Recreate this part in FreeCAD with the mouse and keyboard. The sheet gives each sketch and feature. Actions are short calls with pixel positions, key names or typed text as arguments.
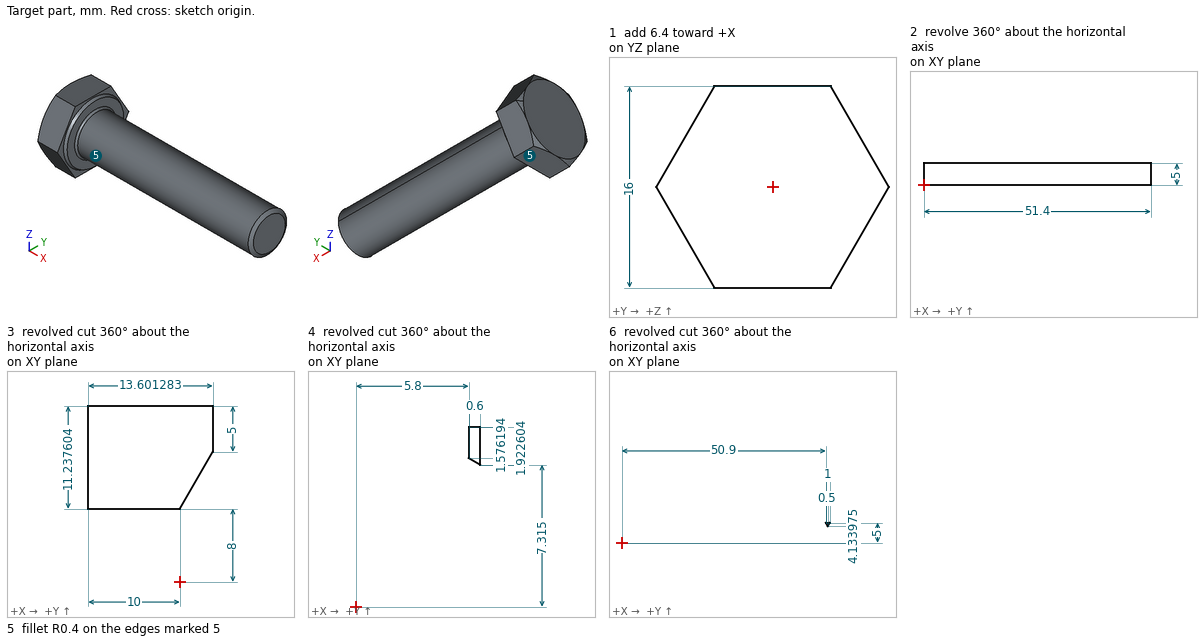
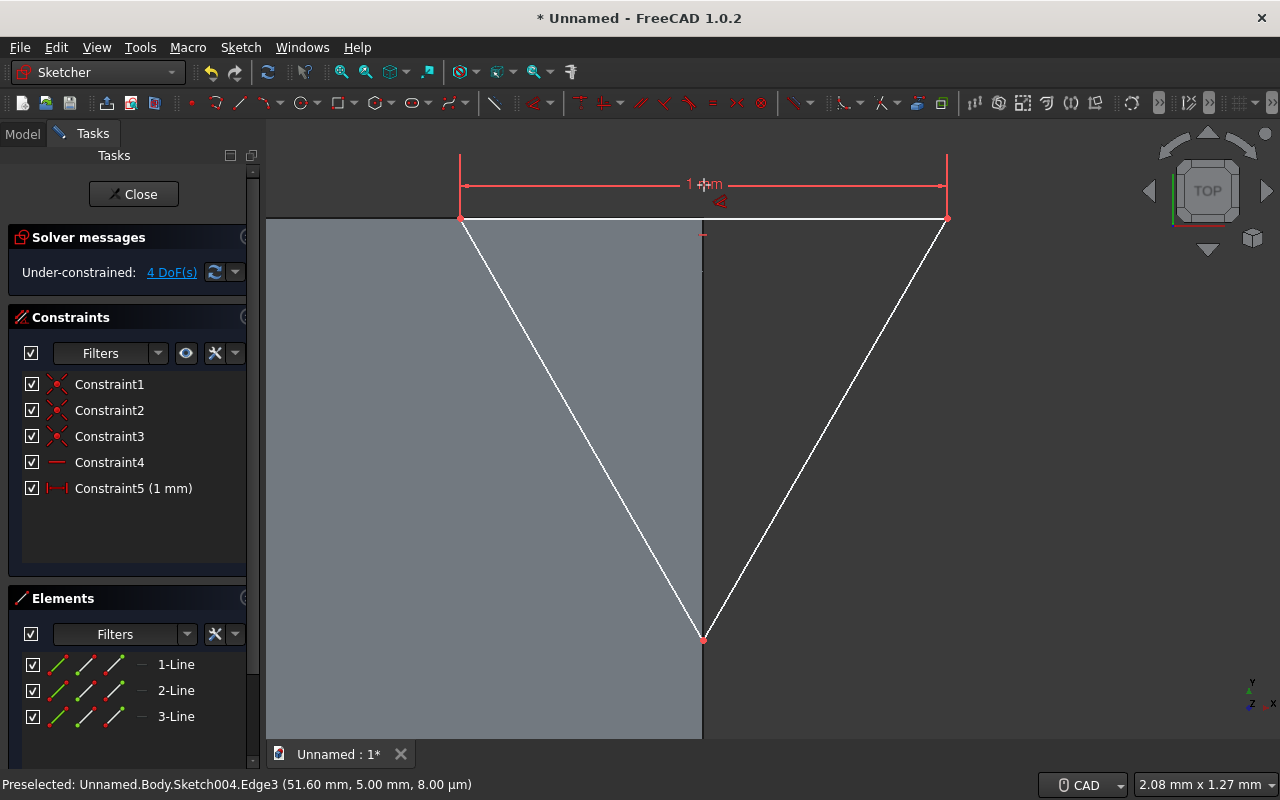
click(460, 219)
click(494, 465)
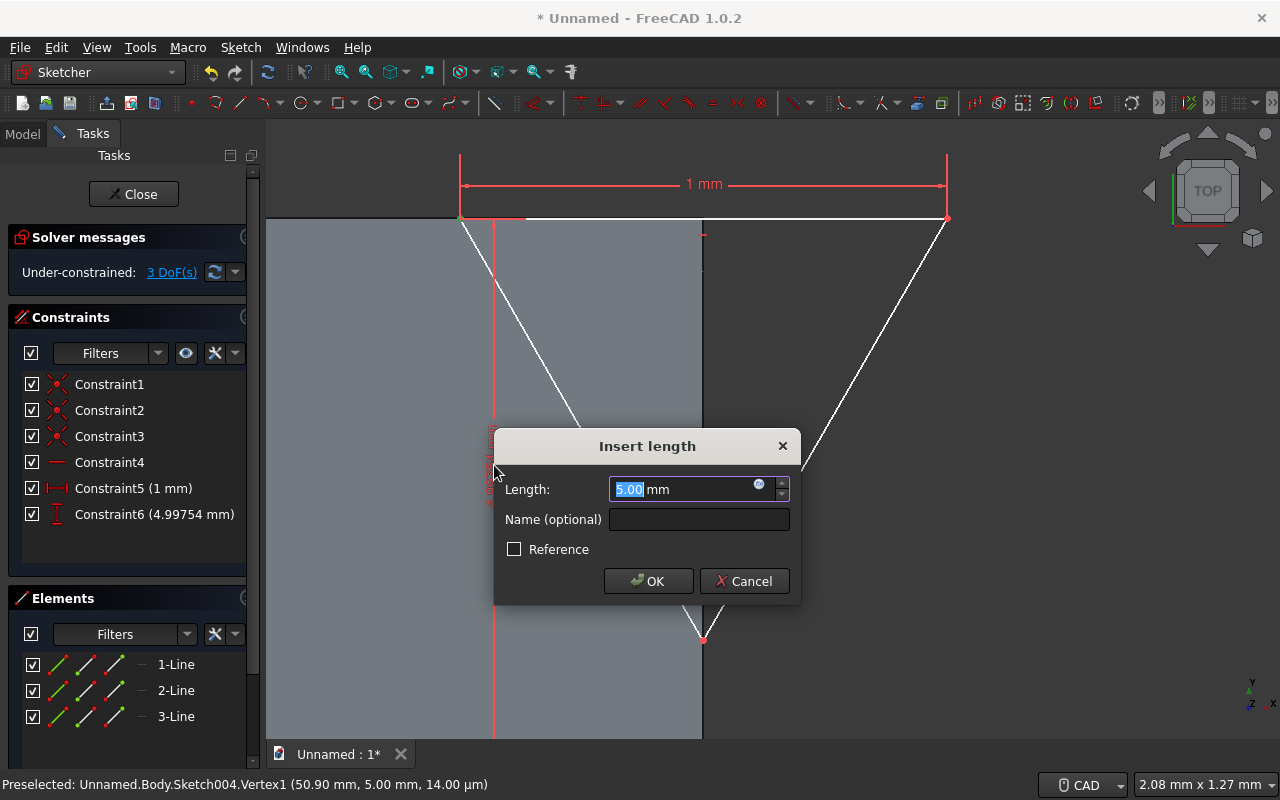
text(5)
key(Return)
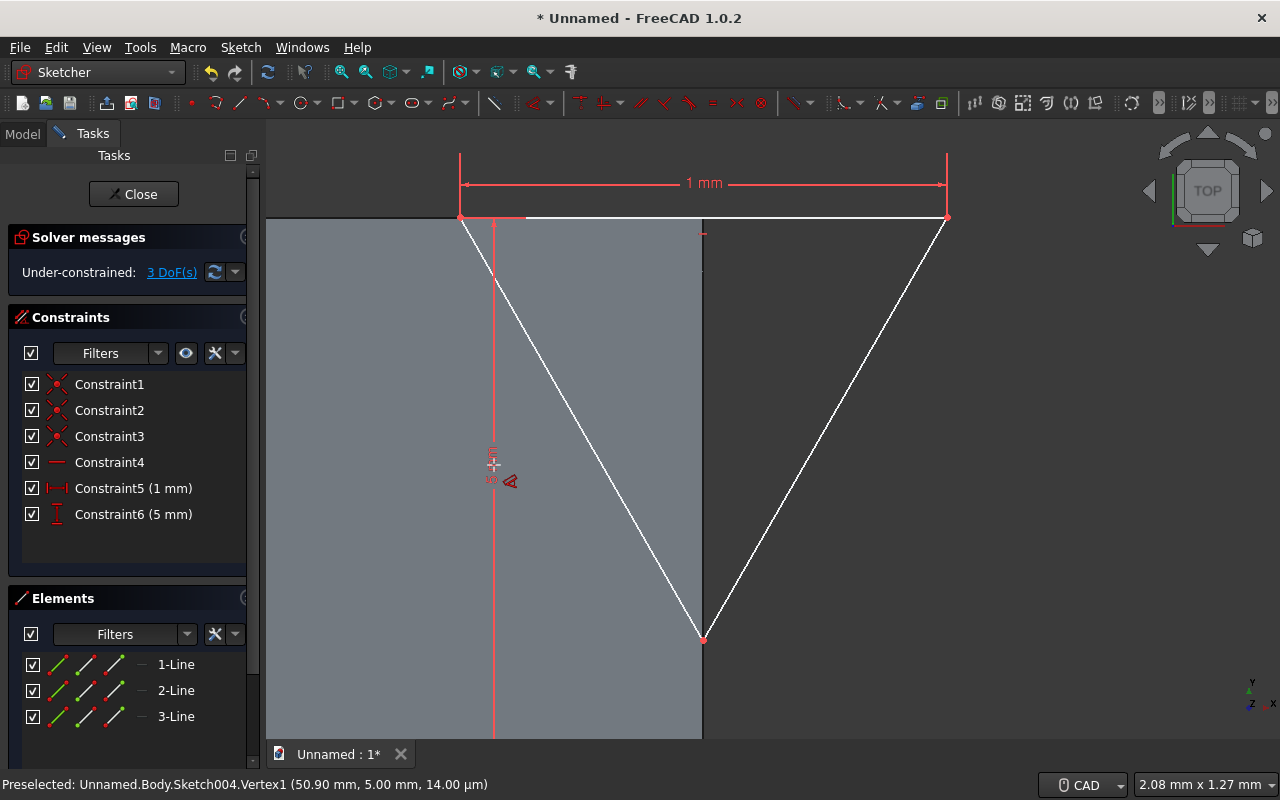
click(533, 345)
click(582, 675)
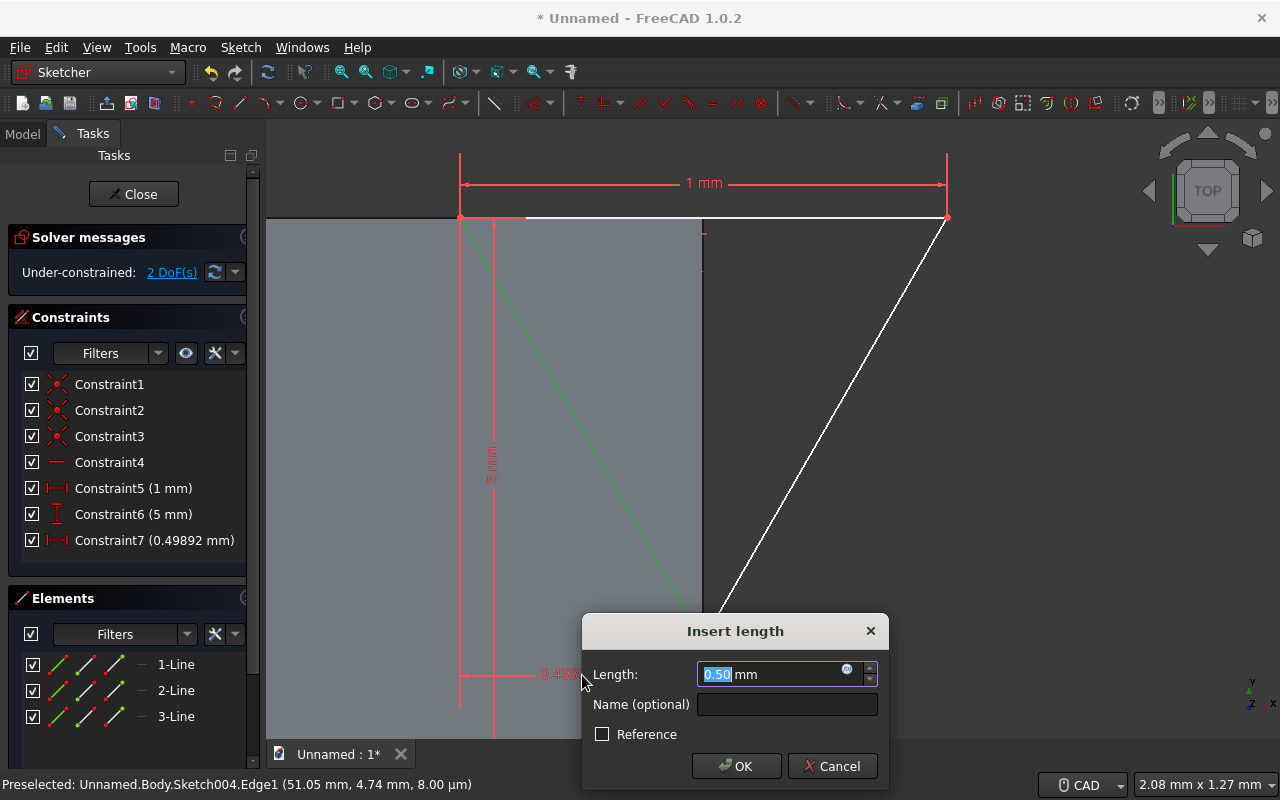
text(0.5)
key(Return)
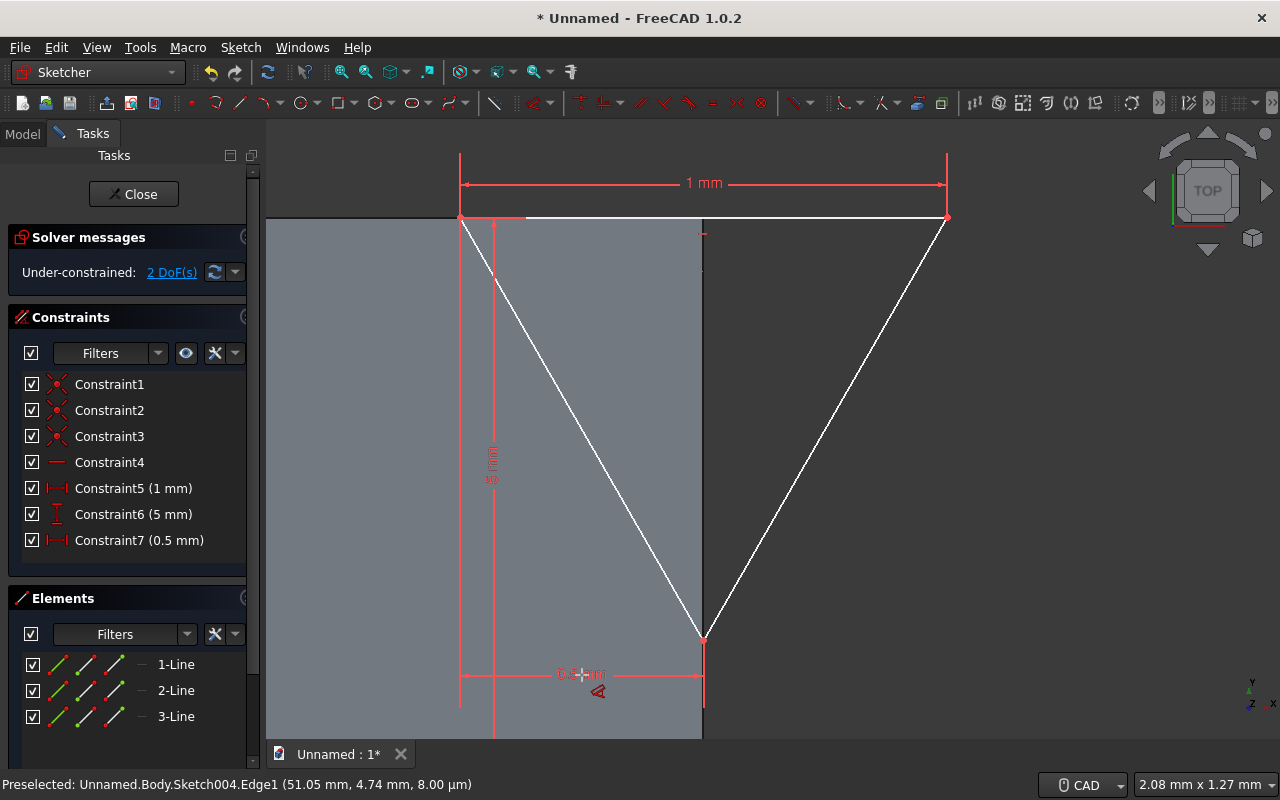
click(460, 218)
click(377, 184)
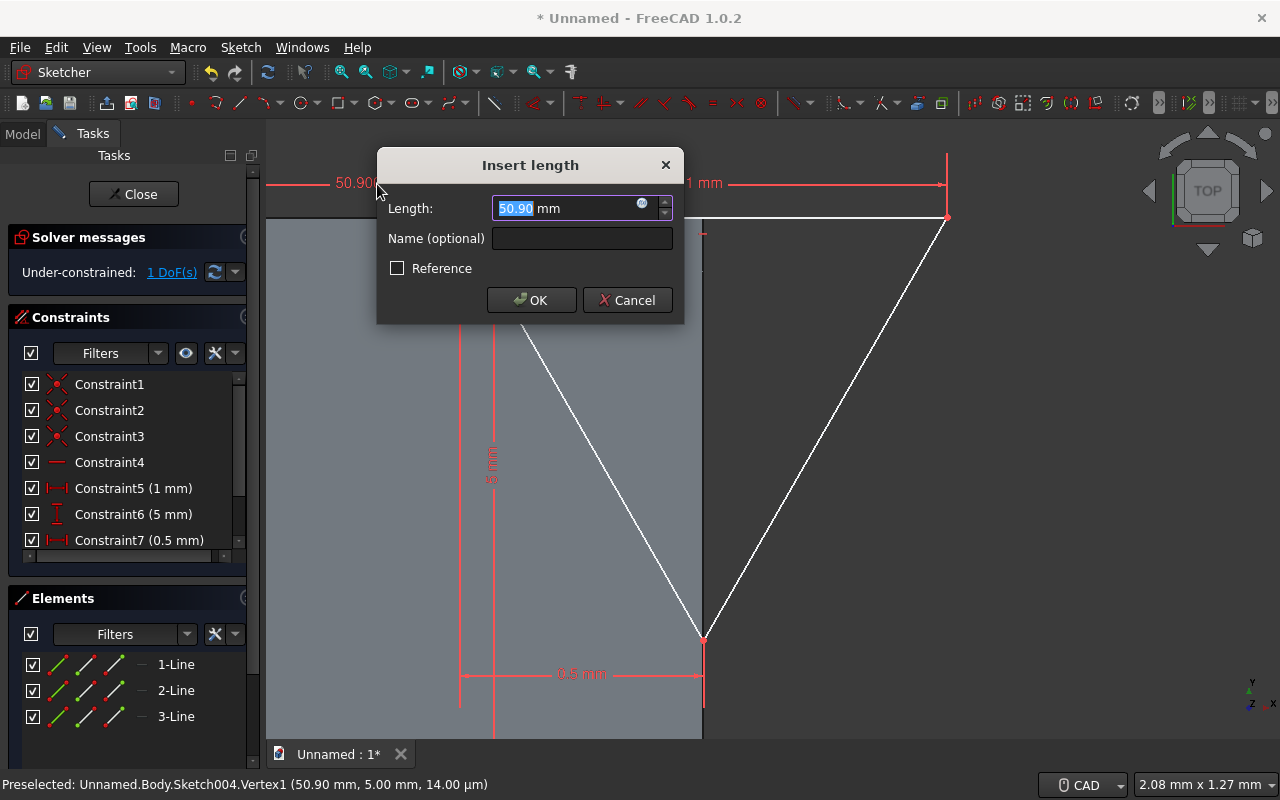
text(50.9)
key(Return)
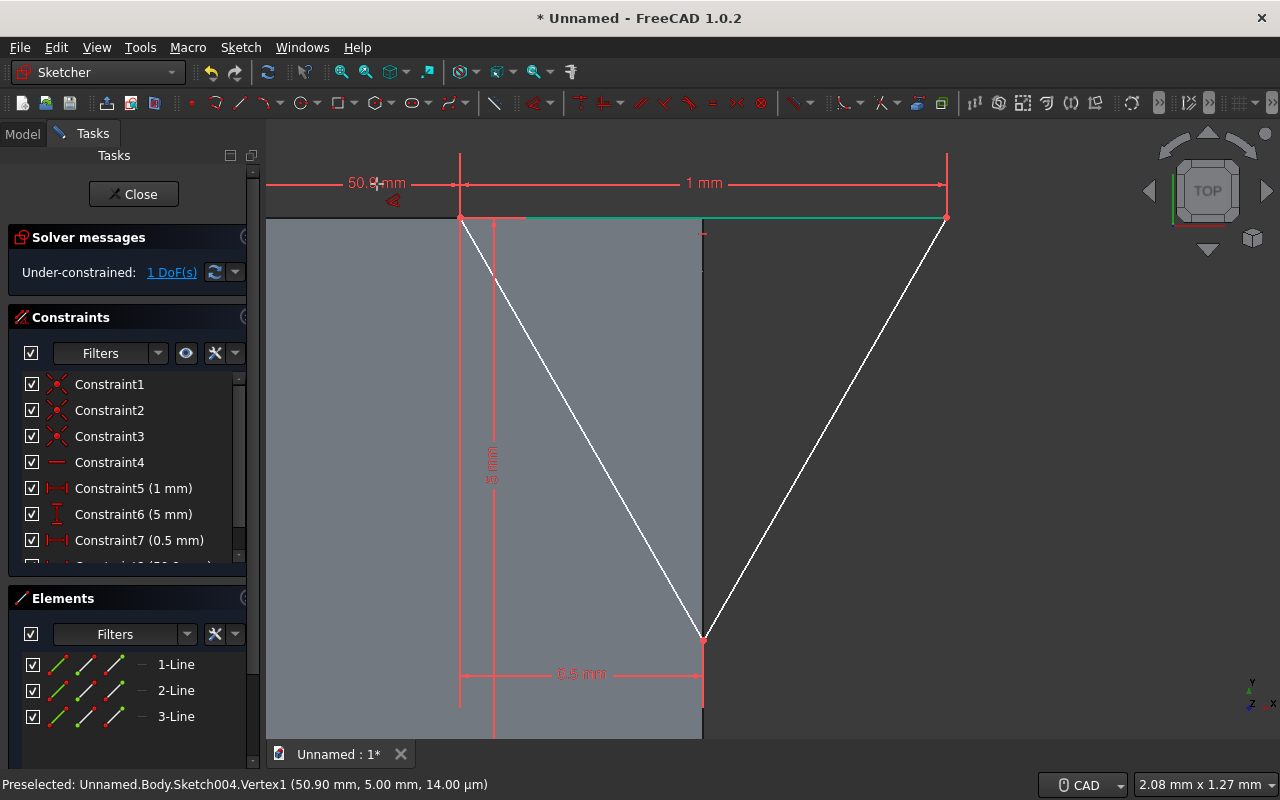
click(703, 641)
click(737, 676)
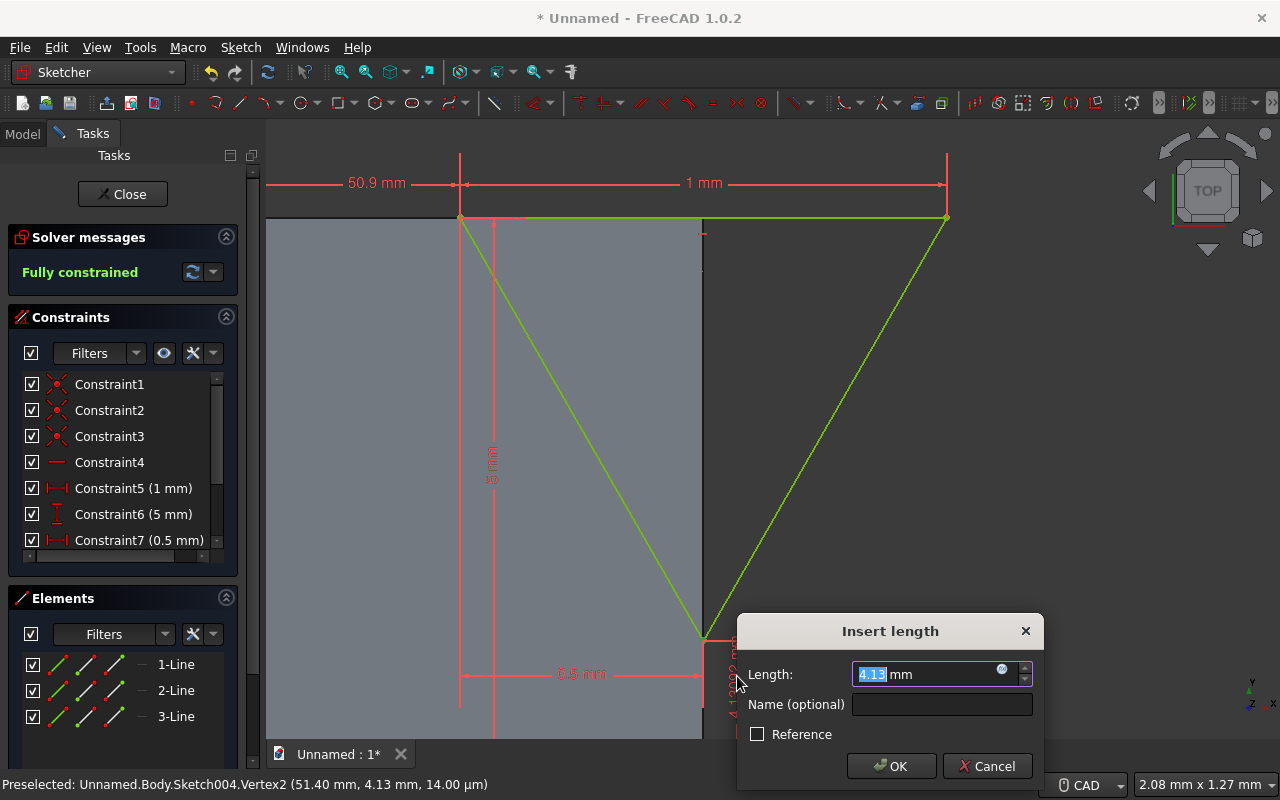
text(4.133975)
key(Return)
key(Escape)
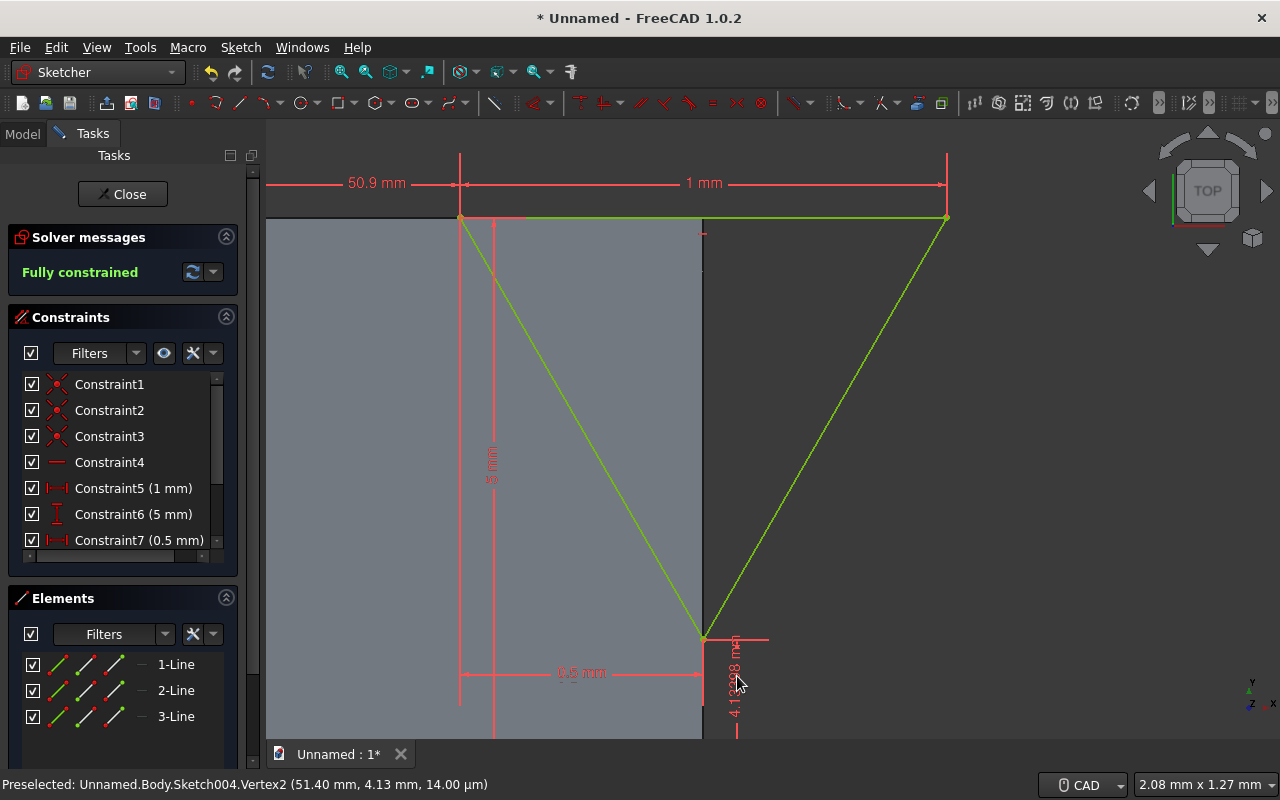
click(123, 194)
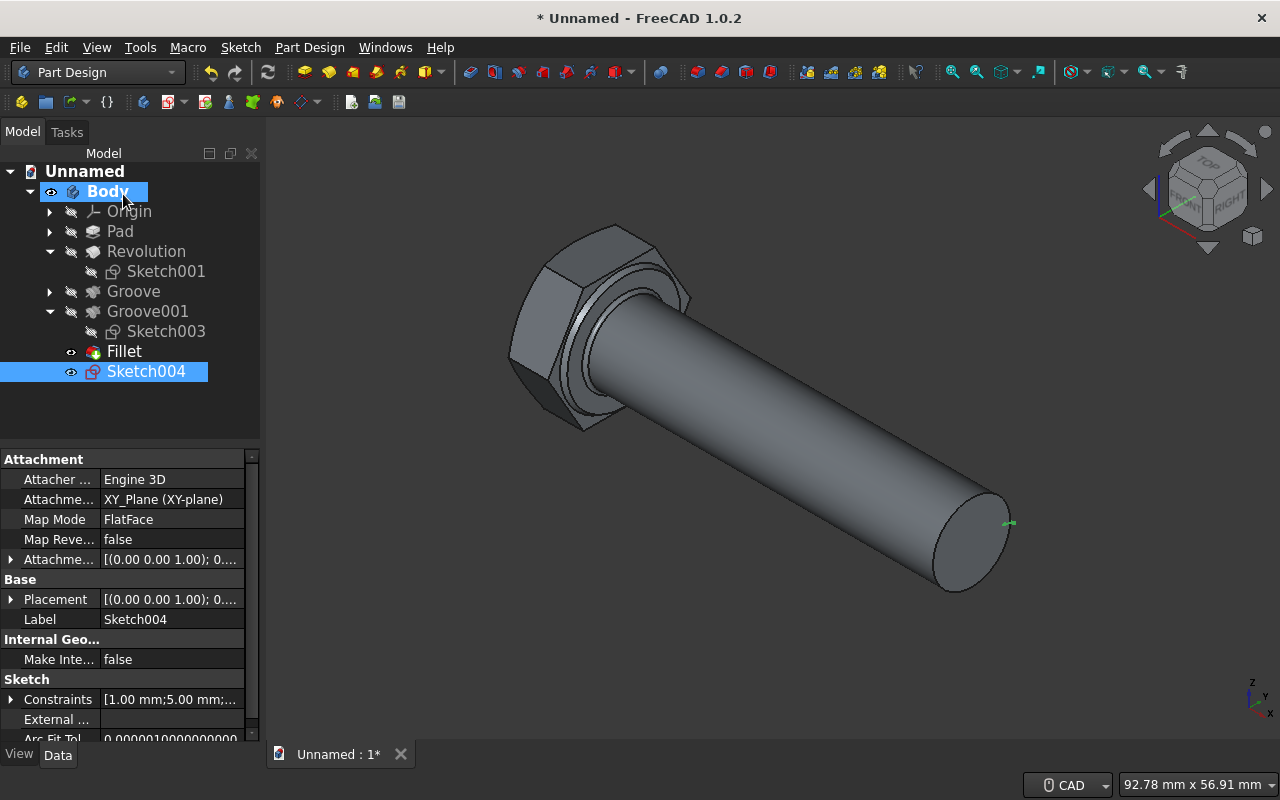
click(520, 72)